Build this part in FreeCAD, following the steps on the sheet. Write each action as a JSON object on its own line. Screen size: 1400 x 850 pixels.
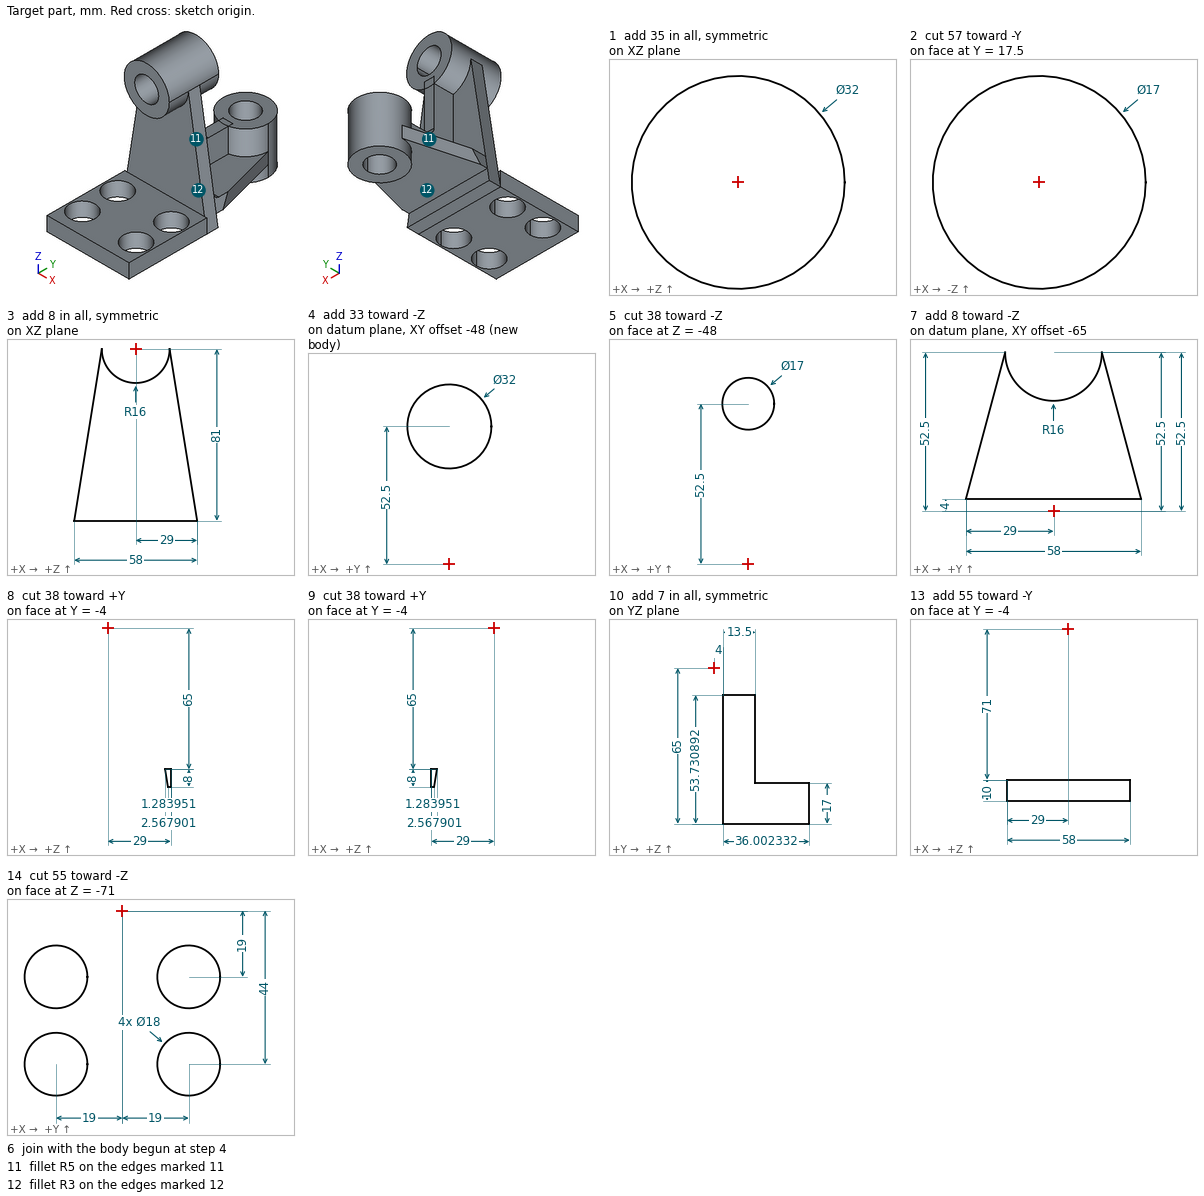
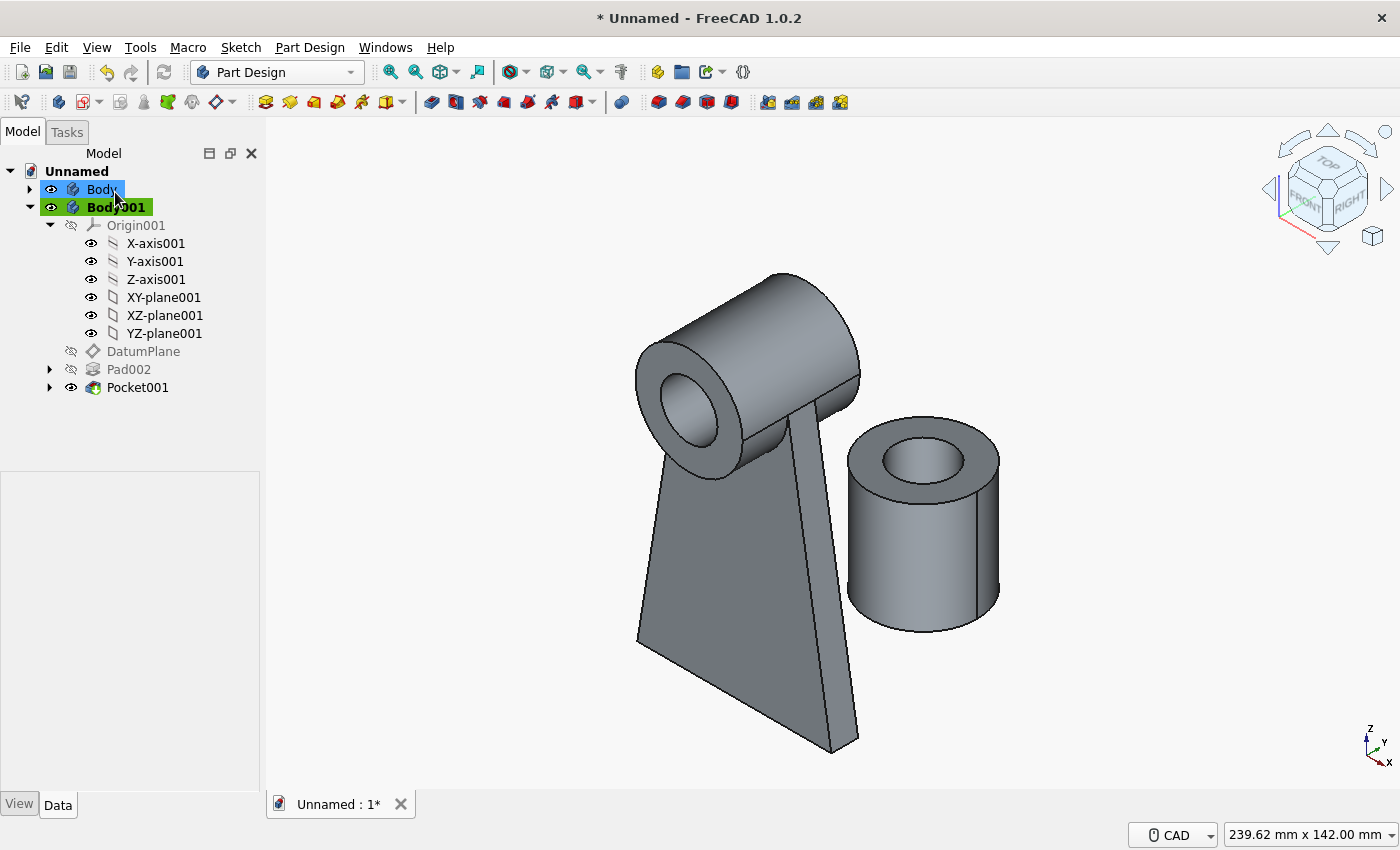
{"action": "key", "text": "v f"}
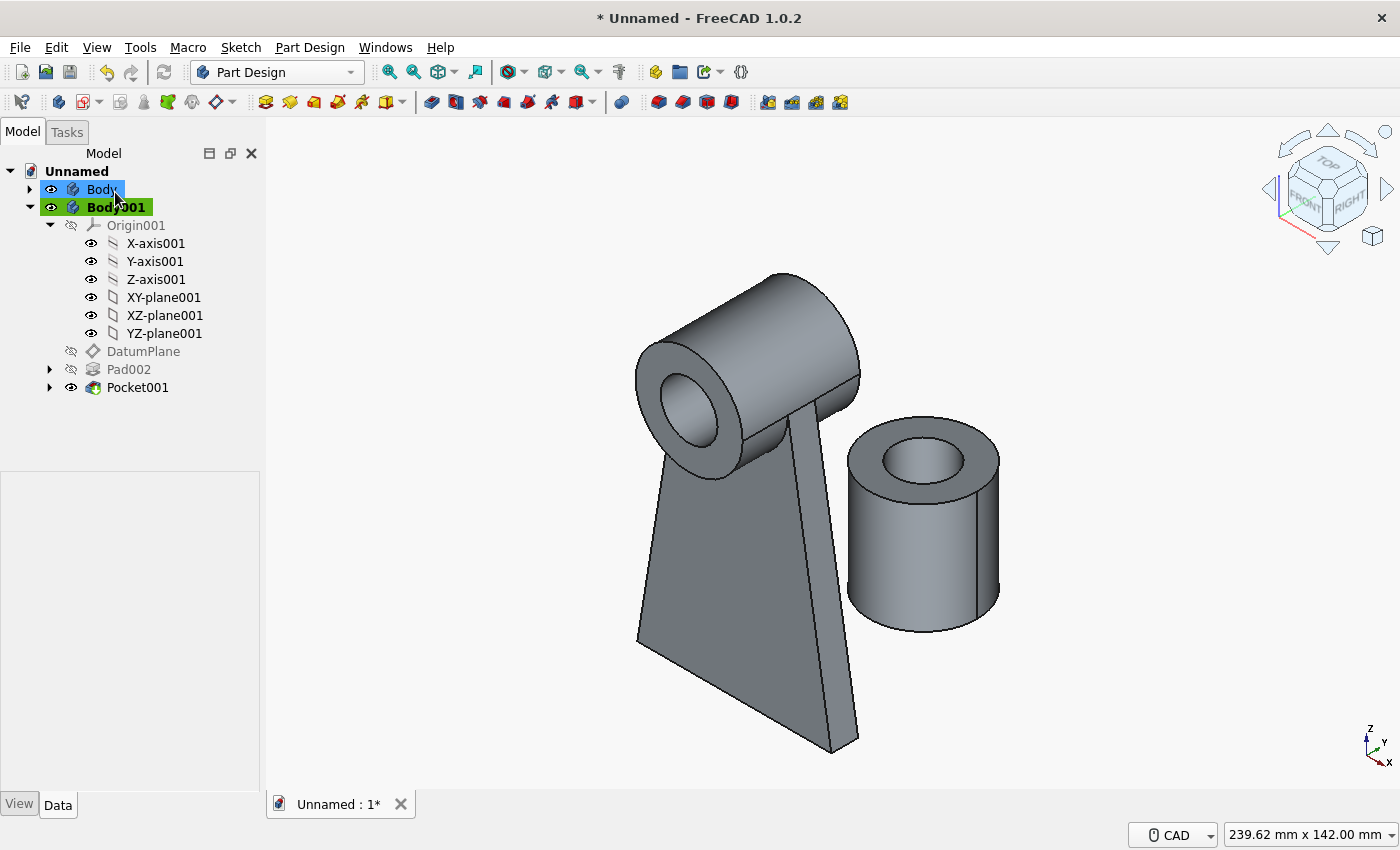
{"action": "double_click", "coordinate": [96, 189]}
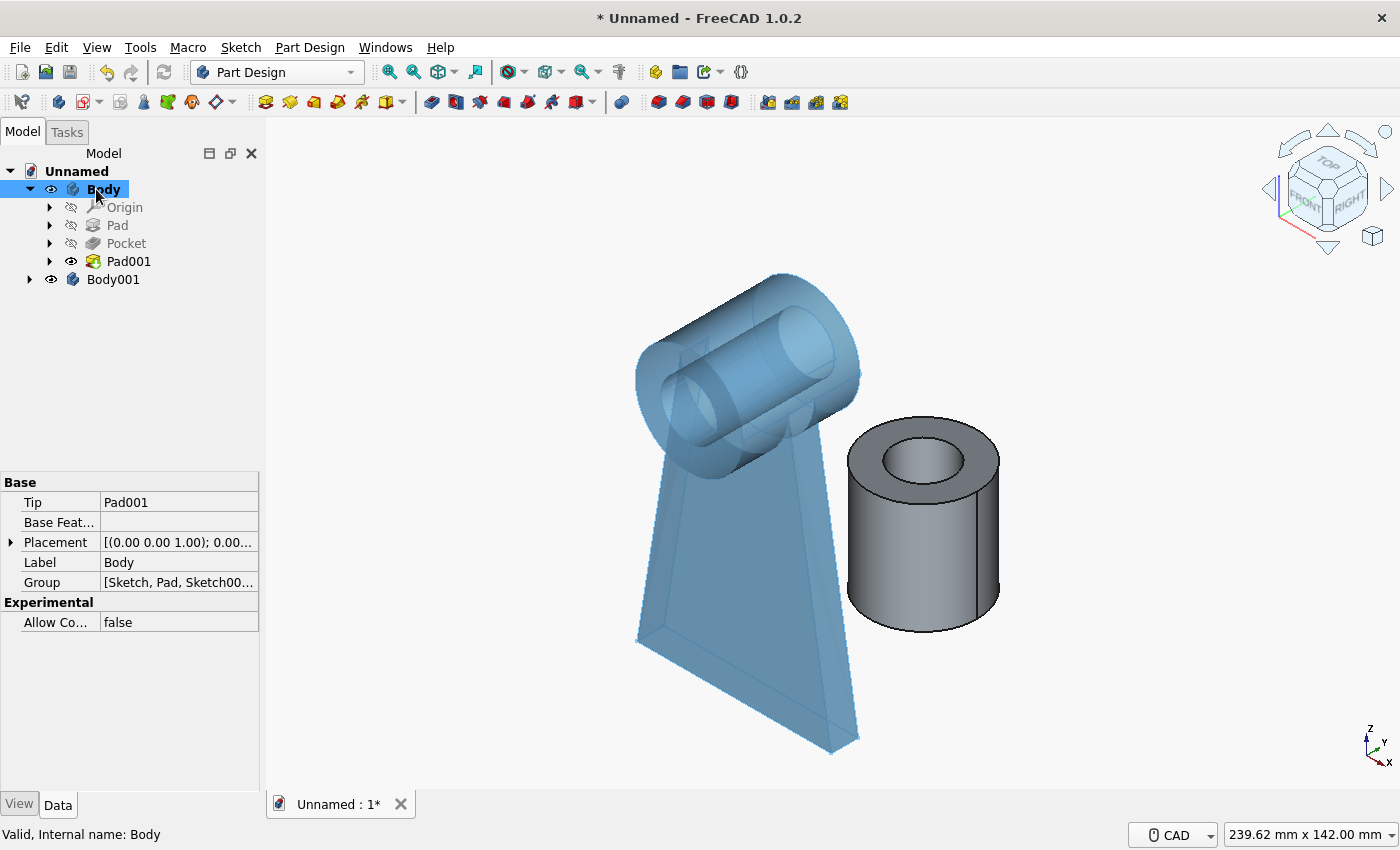
{"action": "left_click", "coordinate": [96, 189]}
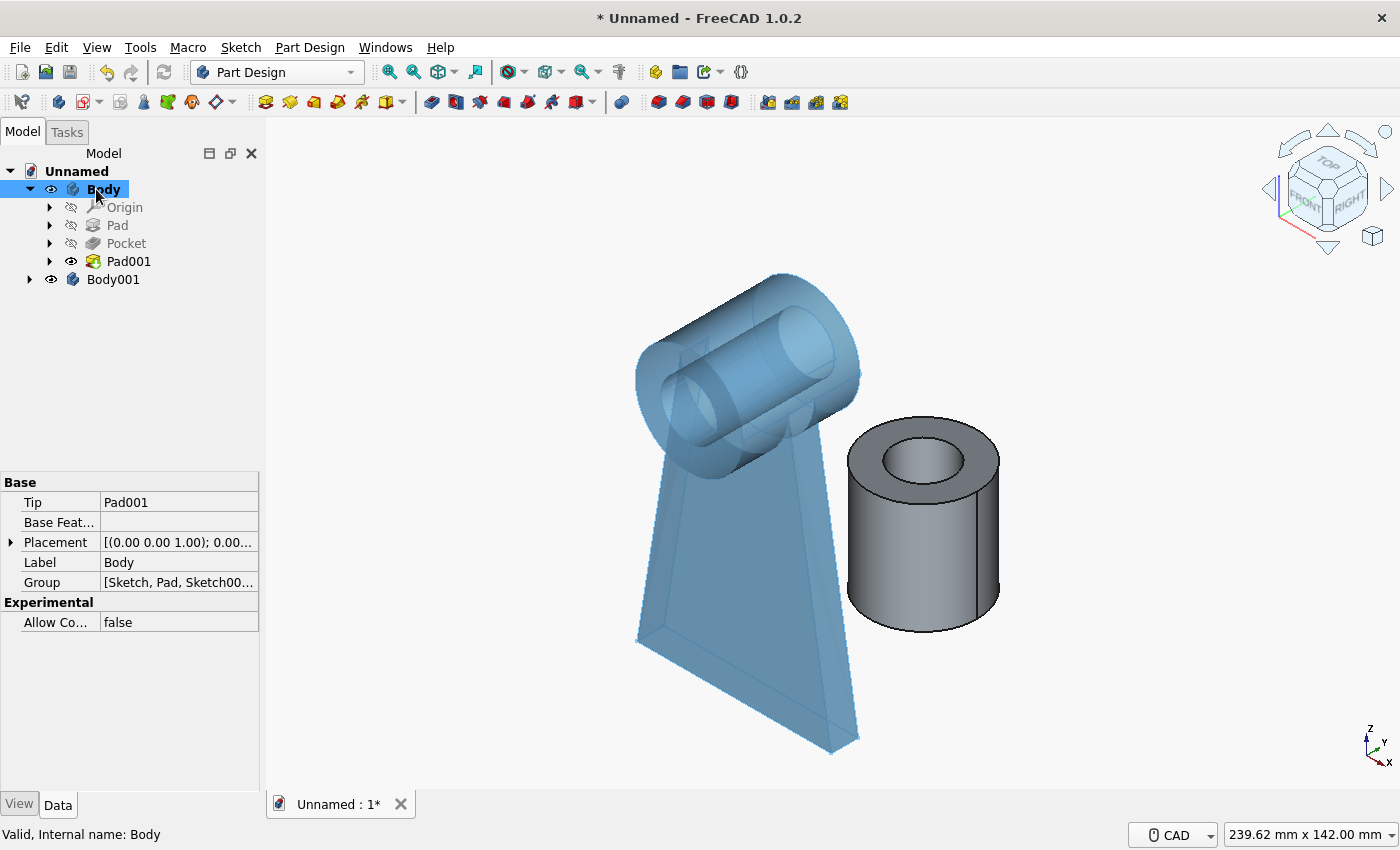
{"action": "left_click", "coordinate": [146, 622]}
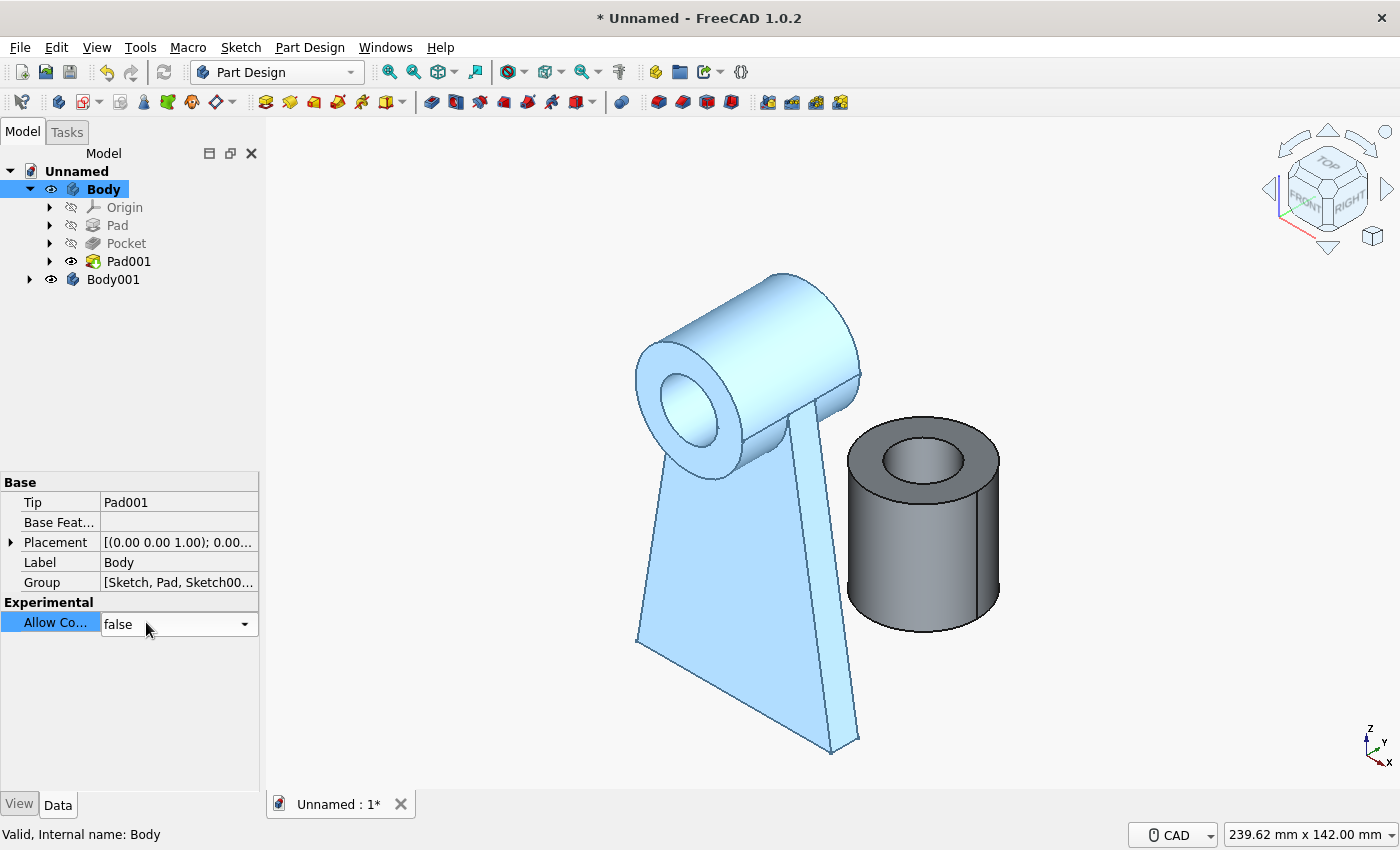
{"action": "left_click", "coordinate": [146, 622]}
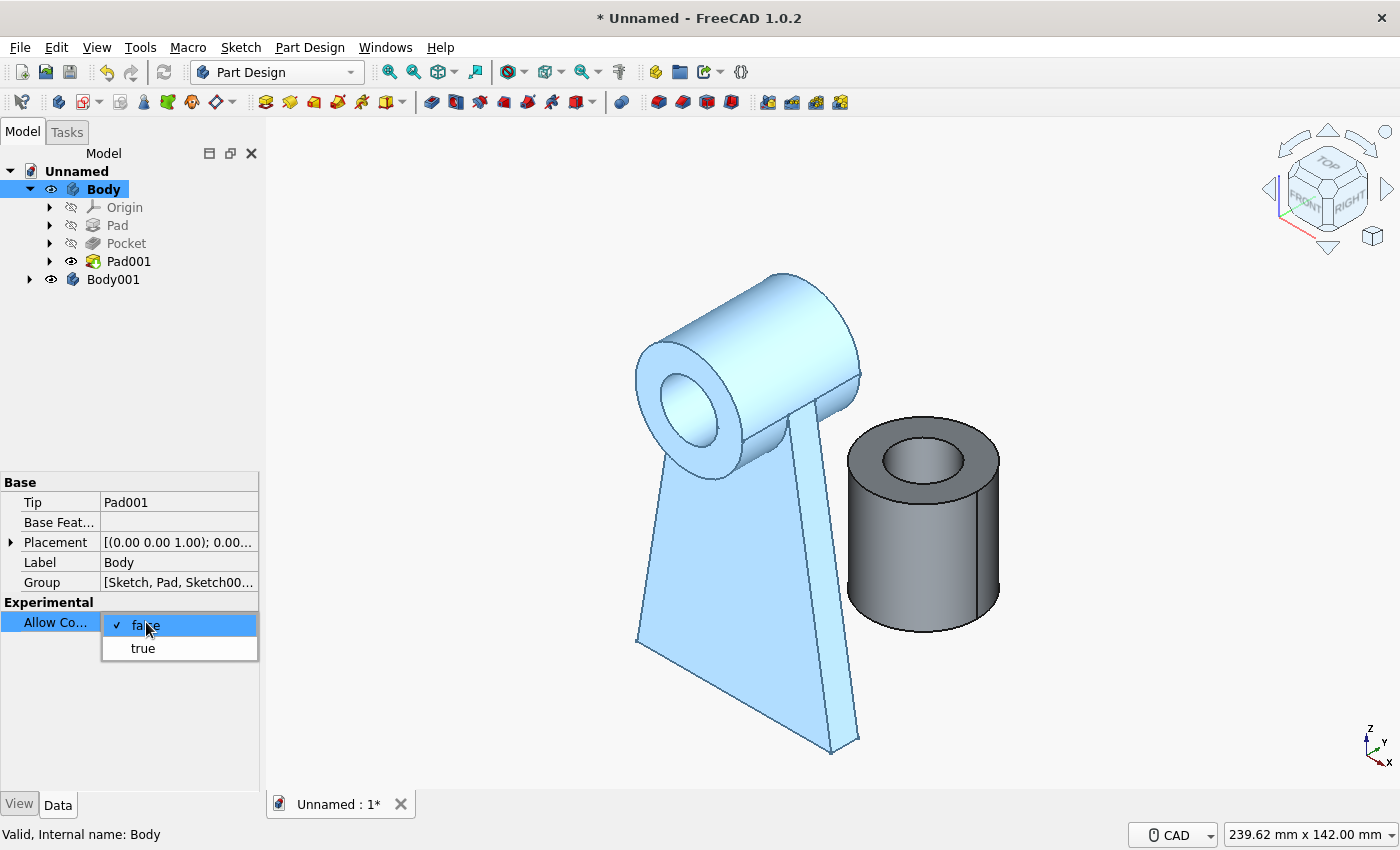
{"action": "left_click", "coordinate": [179, 648]}
{"action": "key", "text": "Return"}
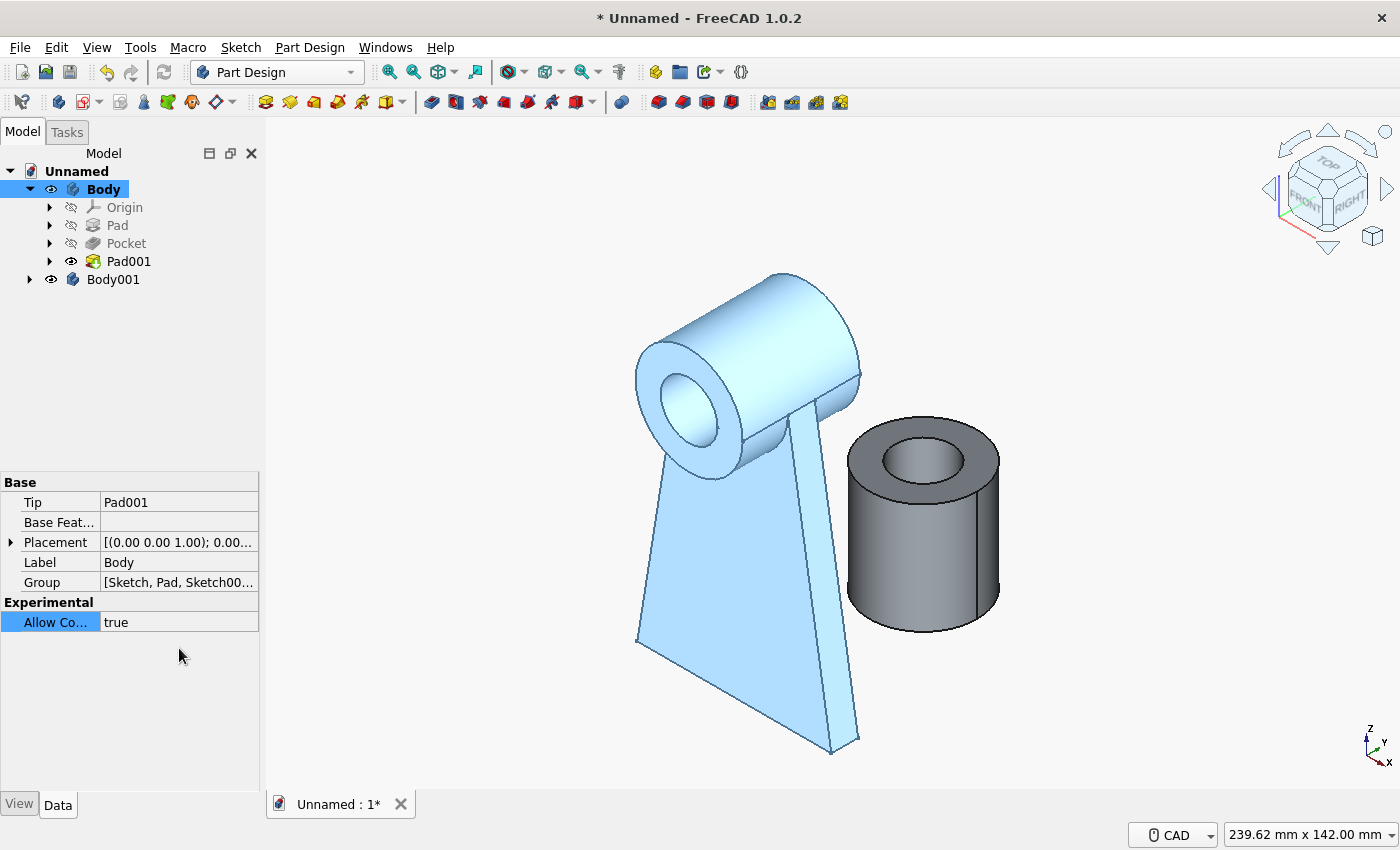
{"action": "left_click", "coordinate": [96, 279]}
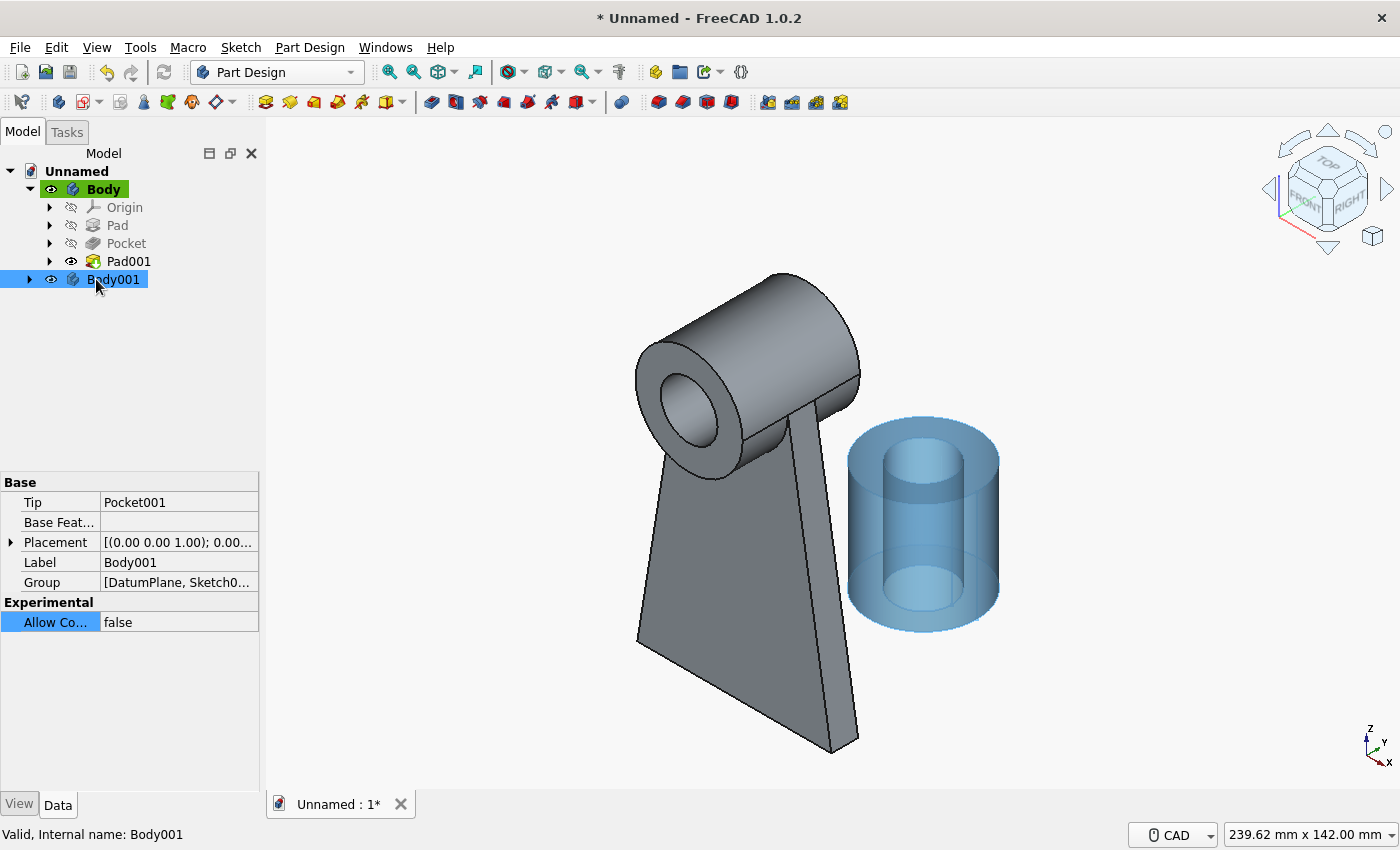
{"action": "left_click", "coordinate": [622, 102]}